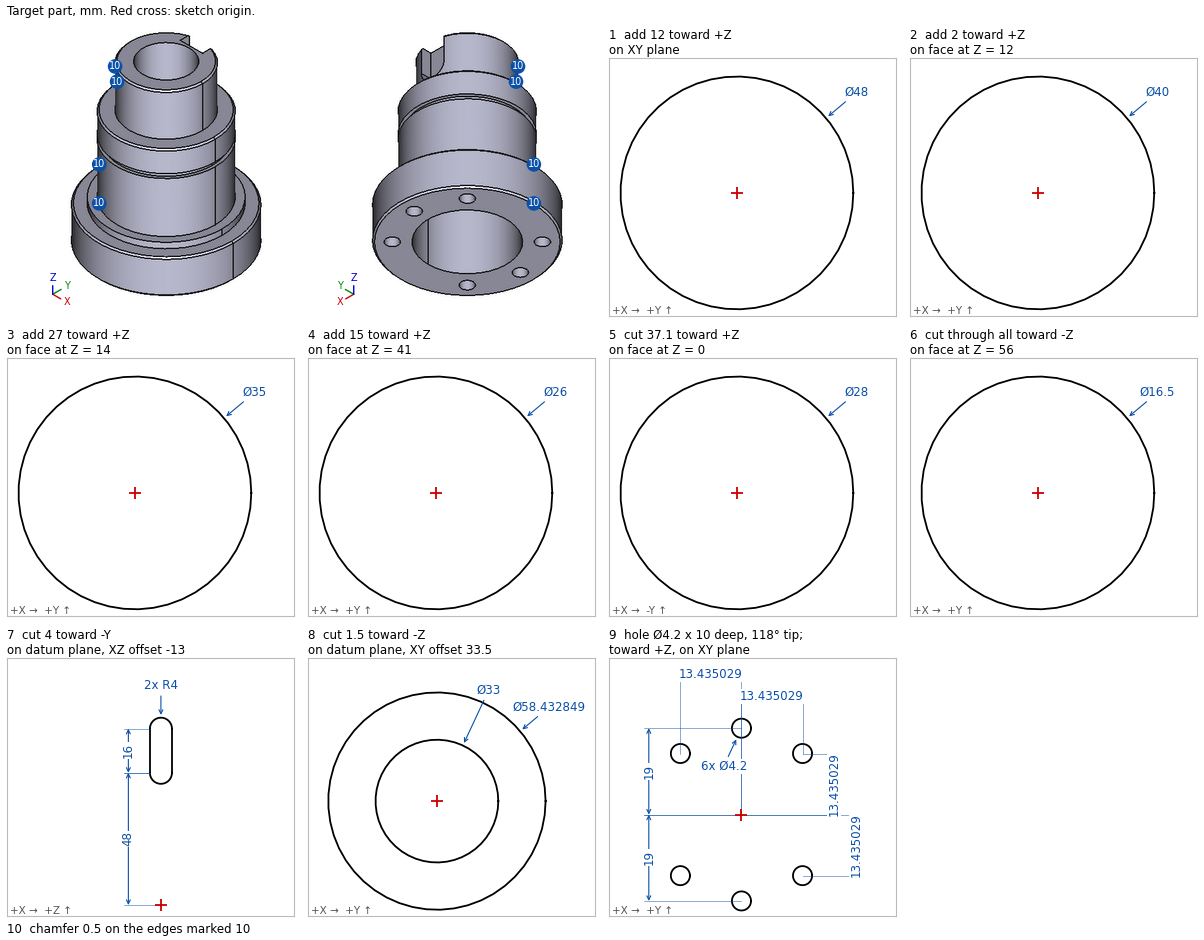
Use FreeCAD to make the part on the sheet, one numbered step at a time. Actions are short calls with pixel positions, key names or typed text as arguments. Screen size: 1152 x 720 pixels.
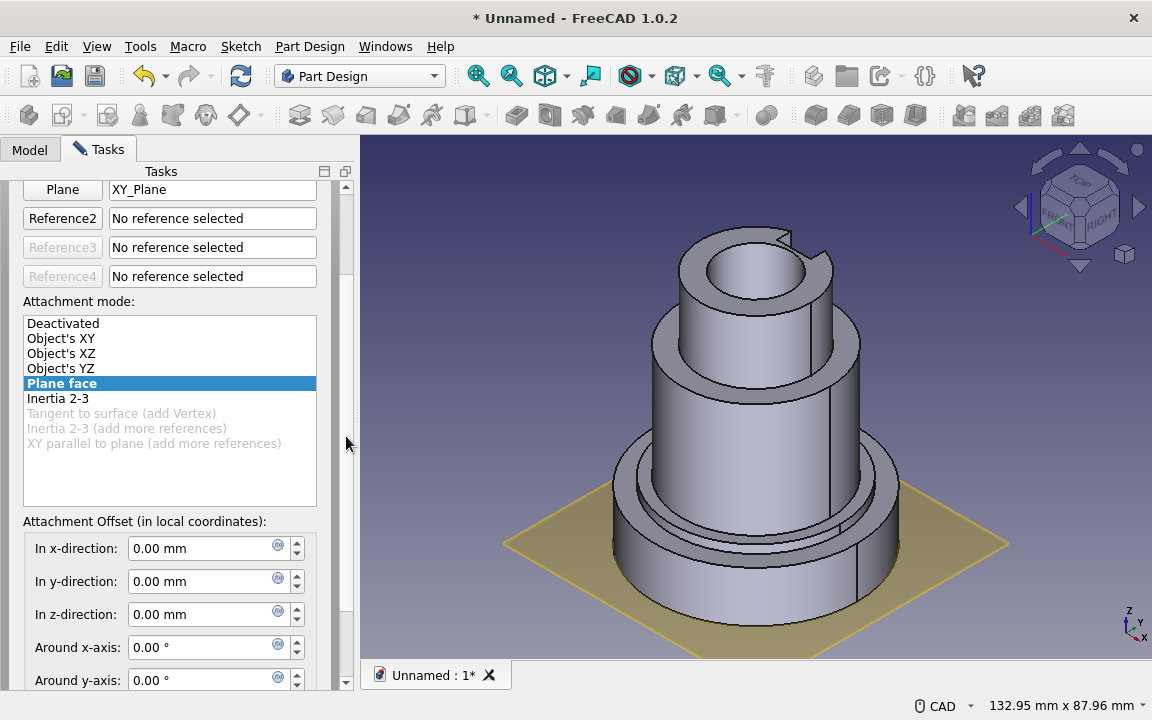
triple_click(210, 614)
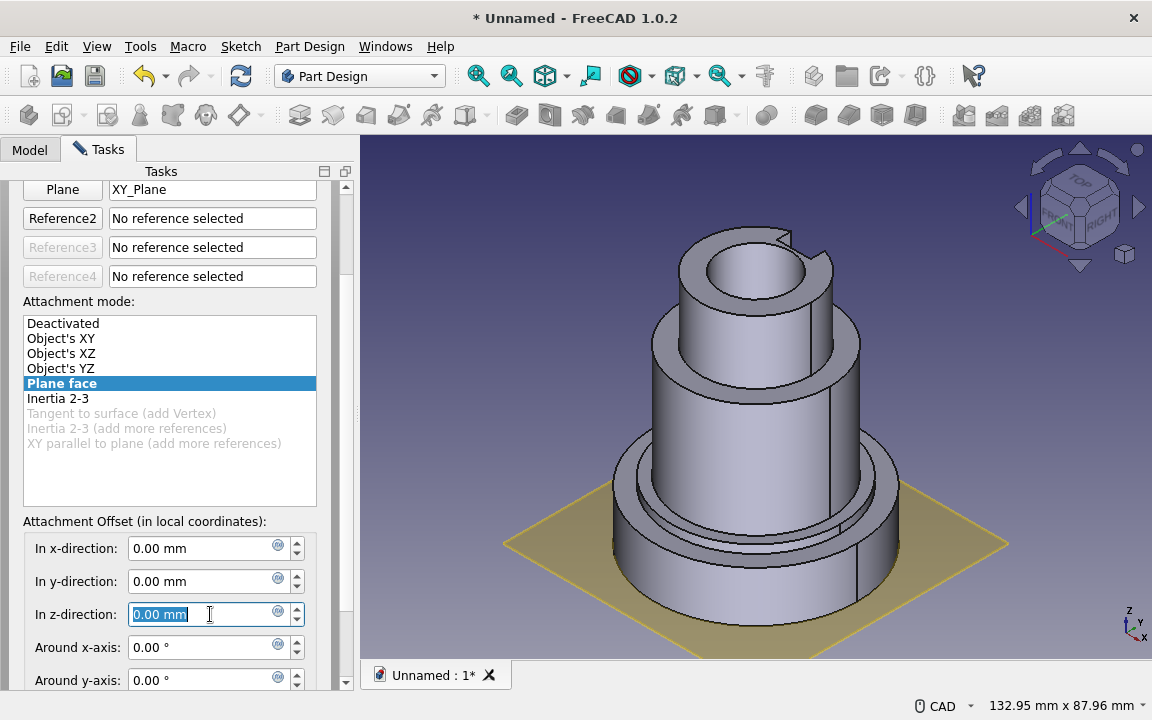
text(33.5)
key(Tab)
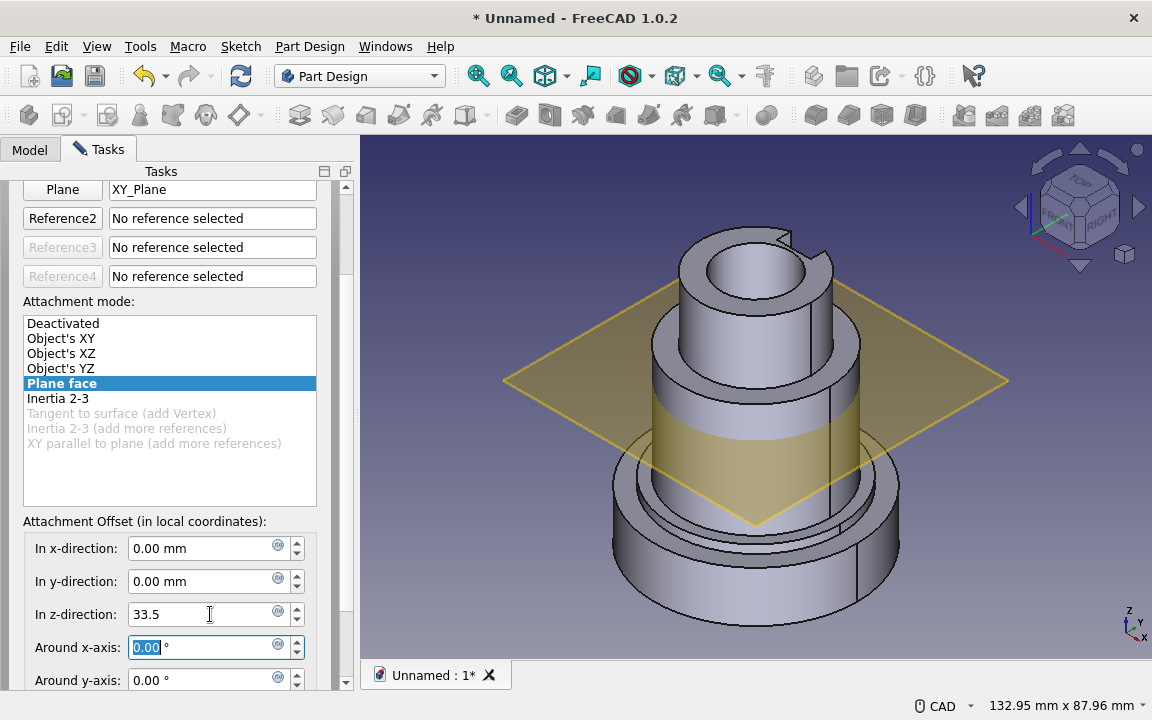
scroll(346, 436, up, 3)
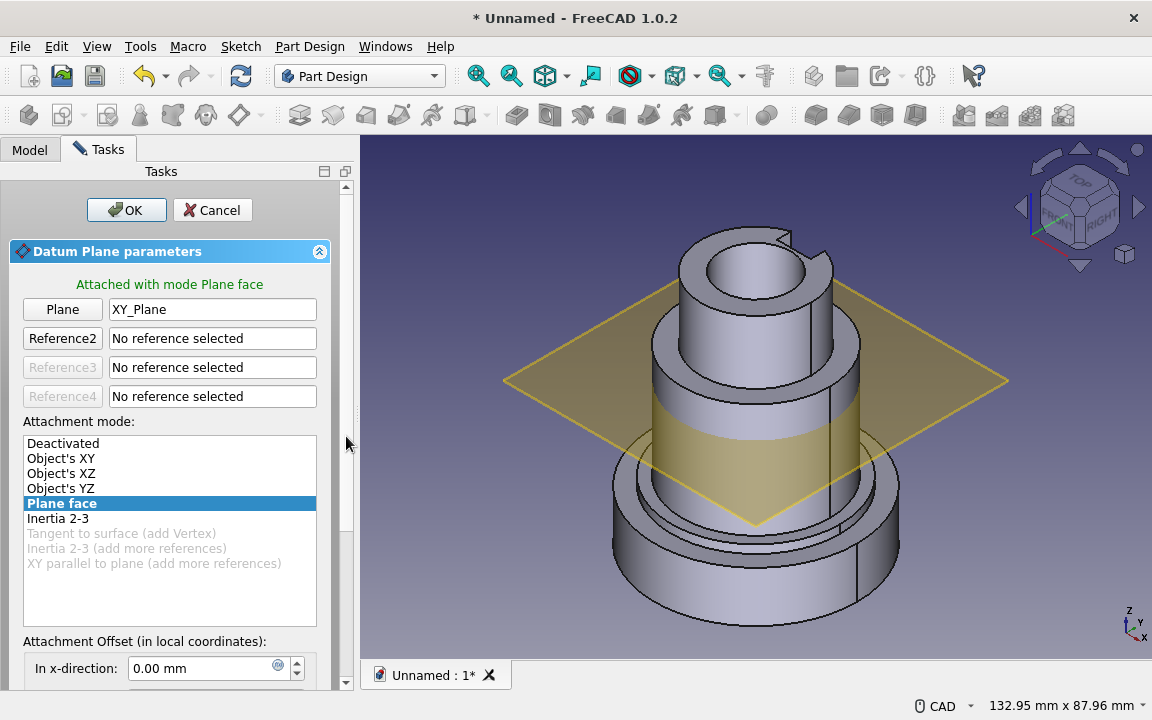
click(127, 210)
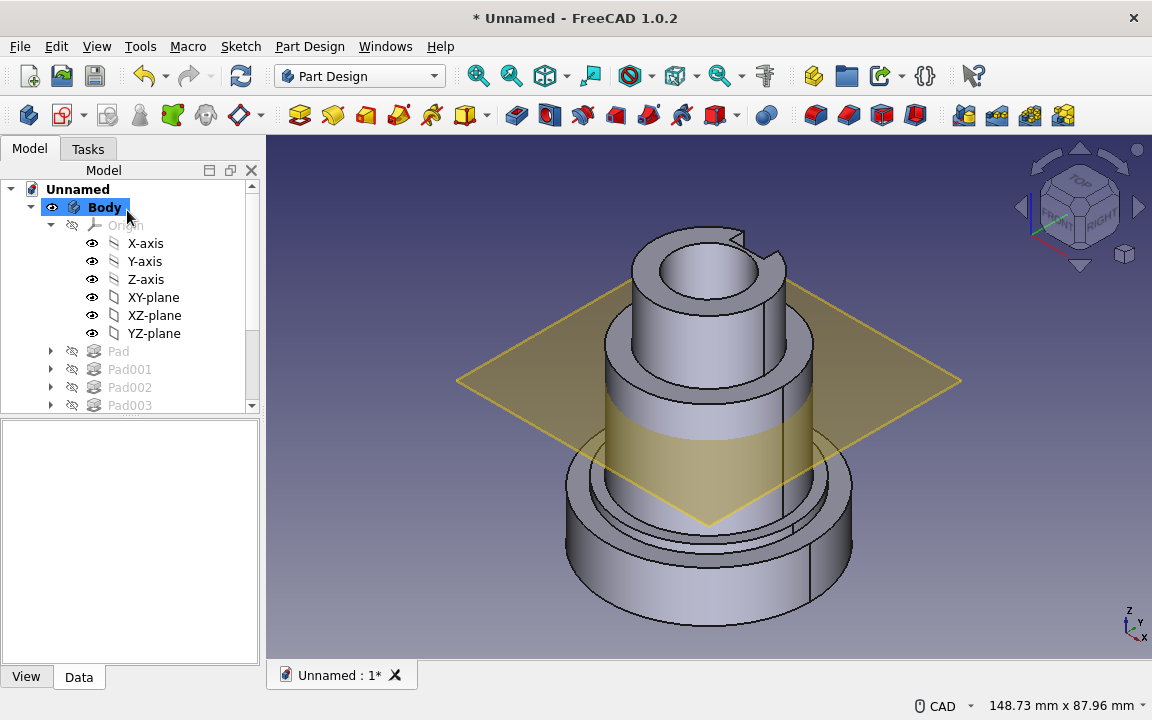
scroll(101, 293, down, 3)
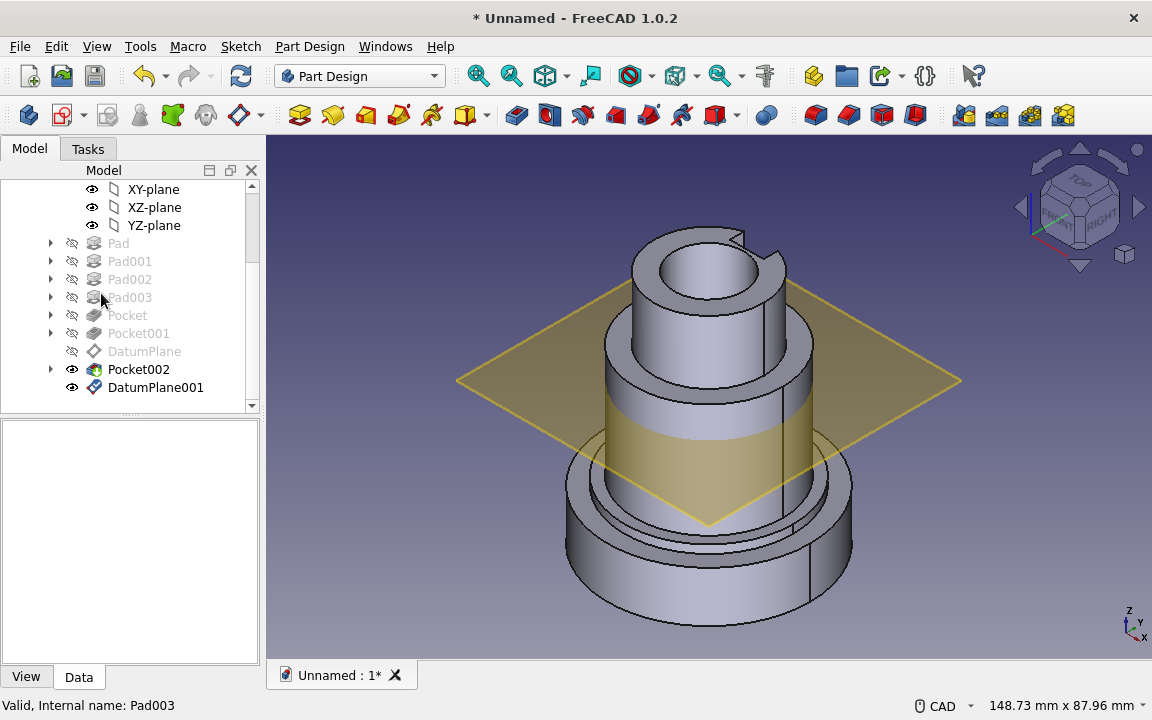
click(117, 387)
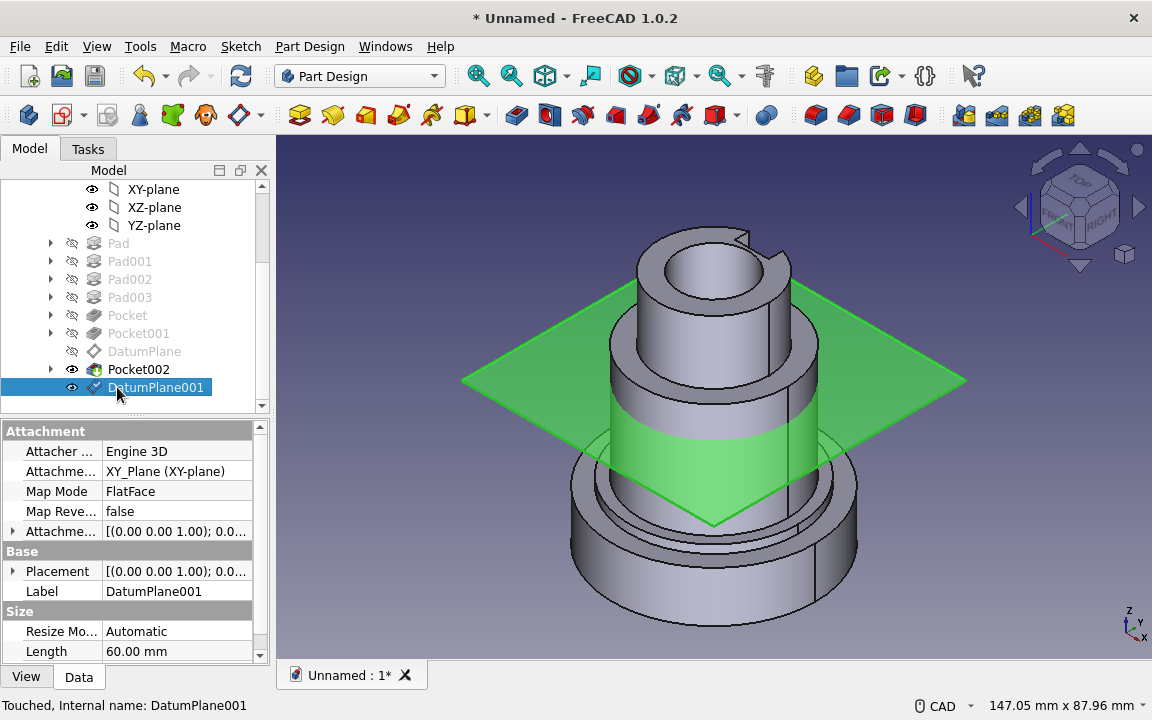
click(62, 116)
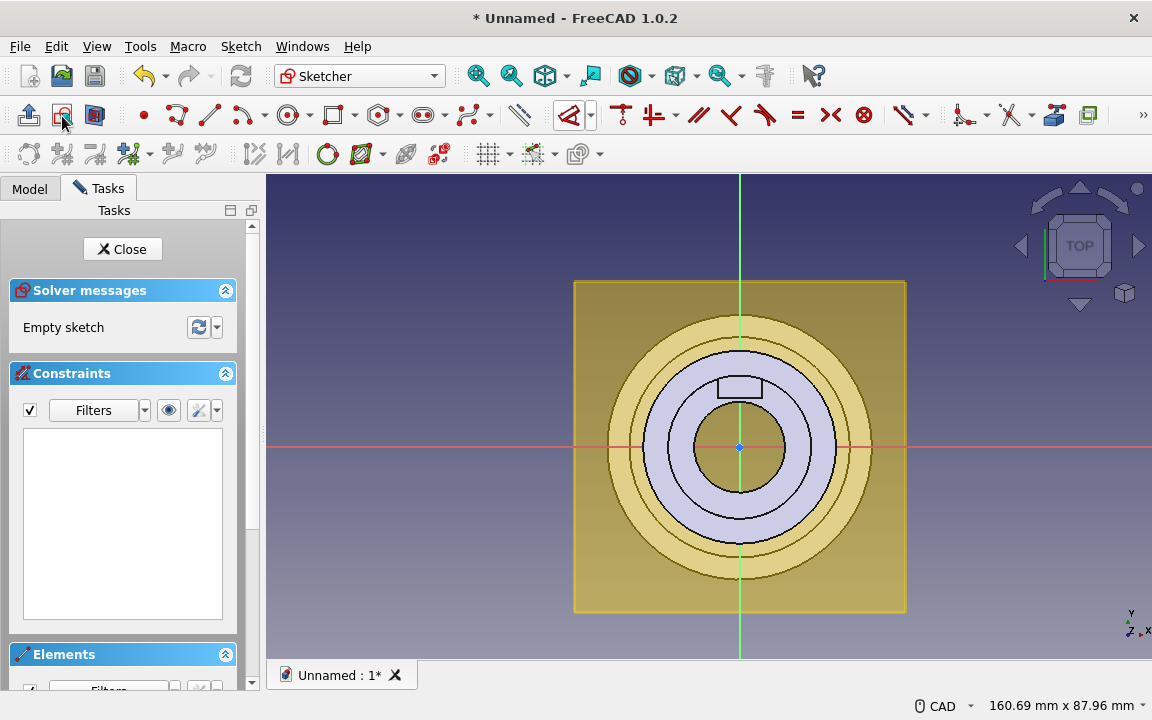
key(q)
key(s)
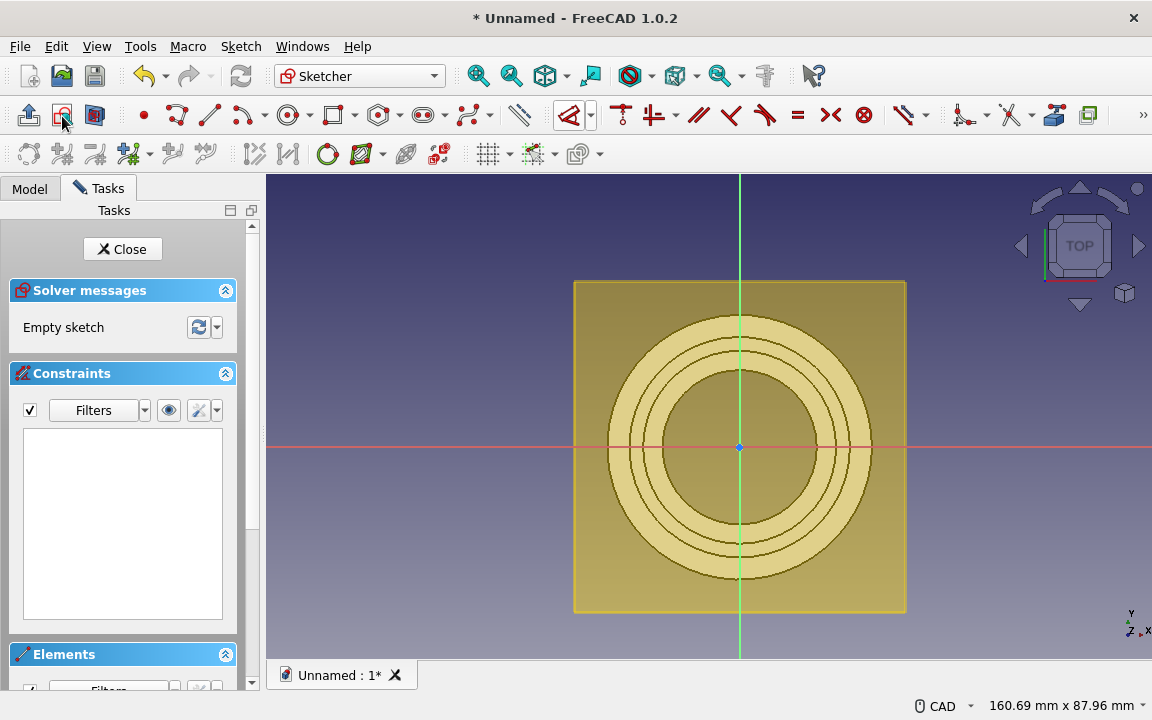
scroll(294, 278, down, 1)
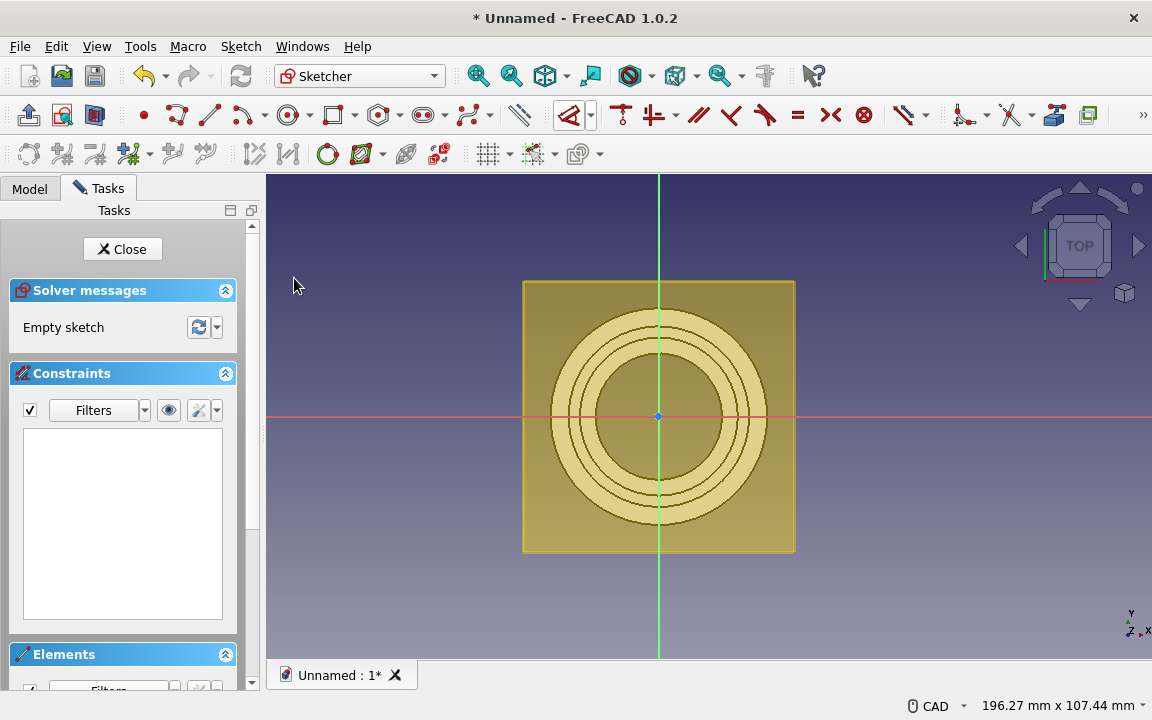
key(g)
key(c)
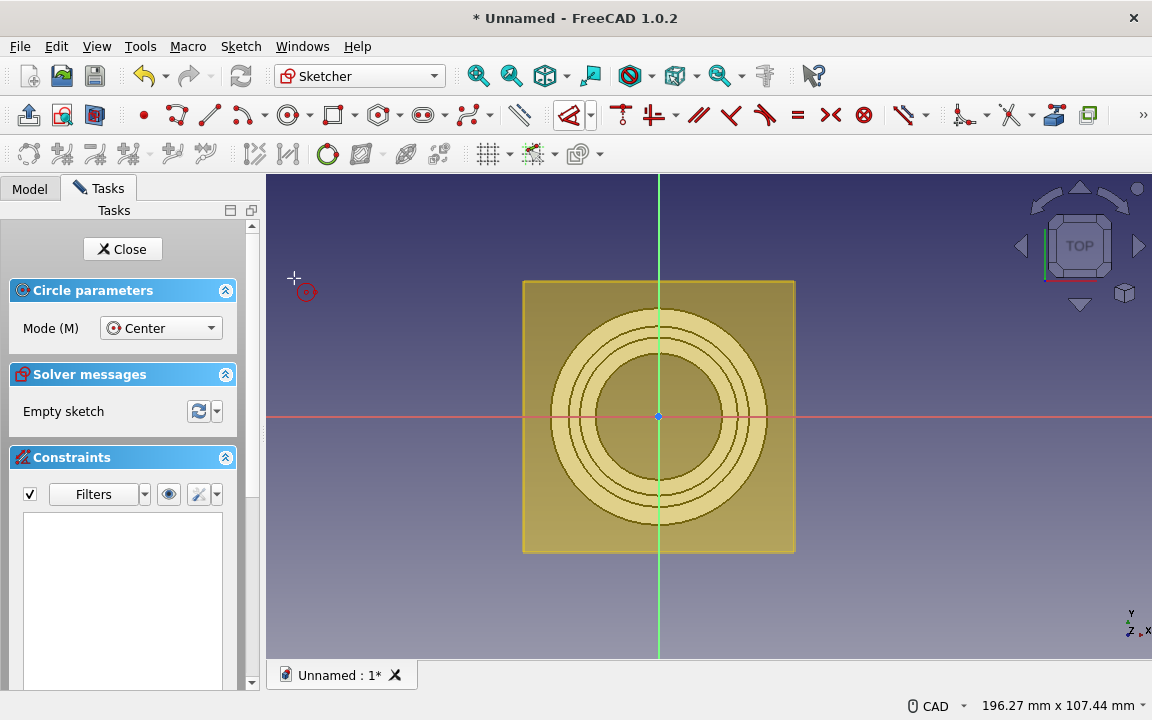
click(659, 417)
click(752, 323)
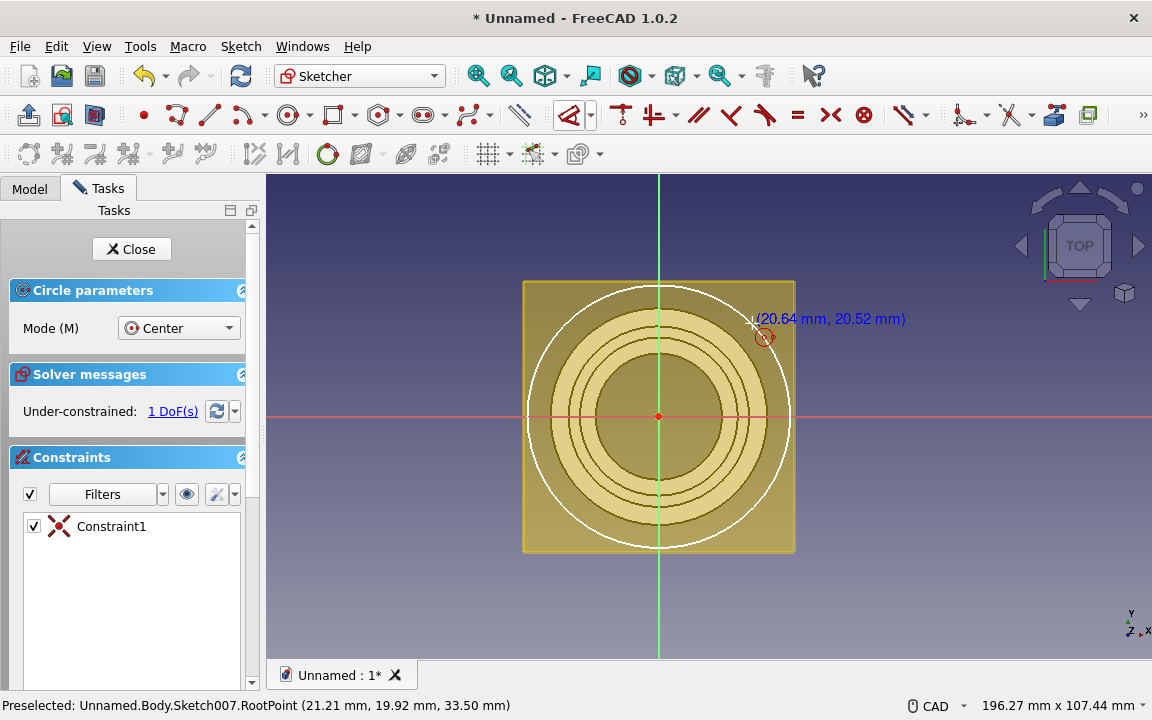
click(659, 417)
click(712, 364)
key(Escape)